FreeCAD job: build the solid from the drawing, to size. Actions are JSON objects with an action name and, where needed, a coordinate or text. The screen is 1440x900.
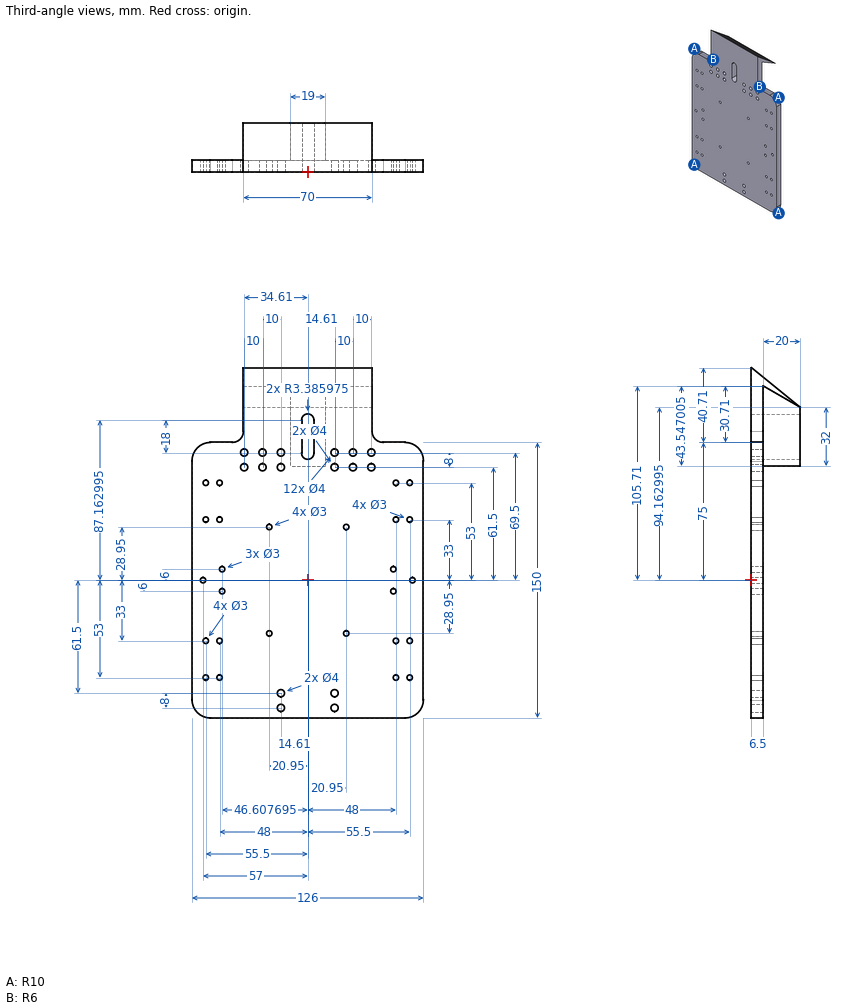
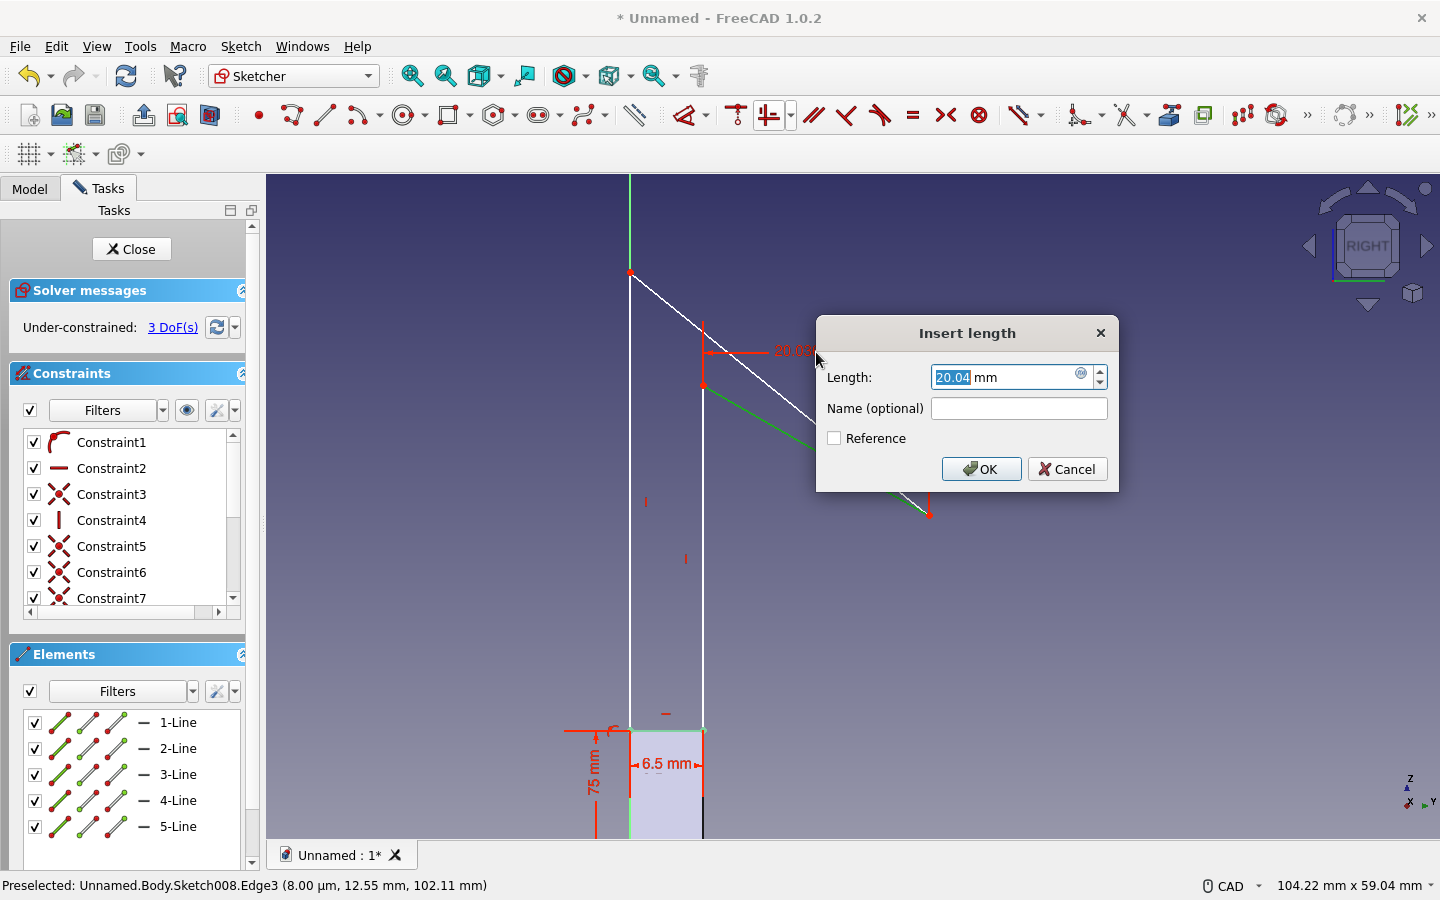
{"action": "type", "text": "20"}
{"action": "key", "text": "Return"}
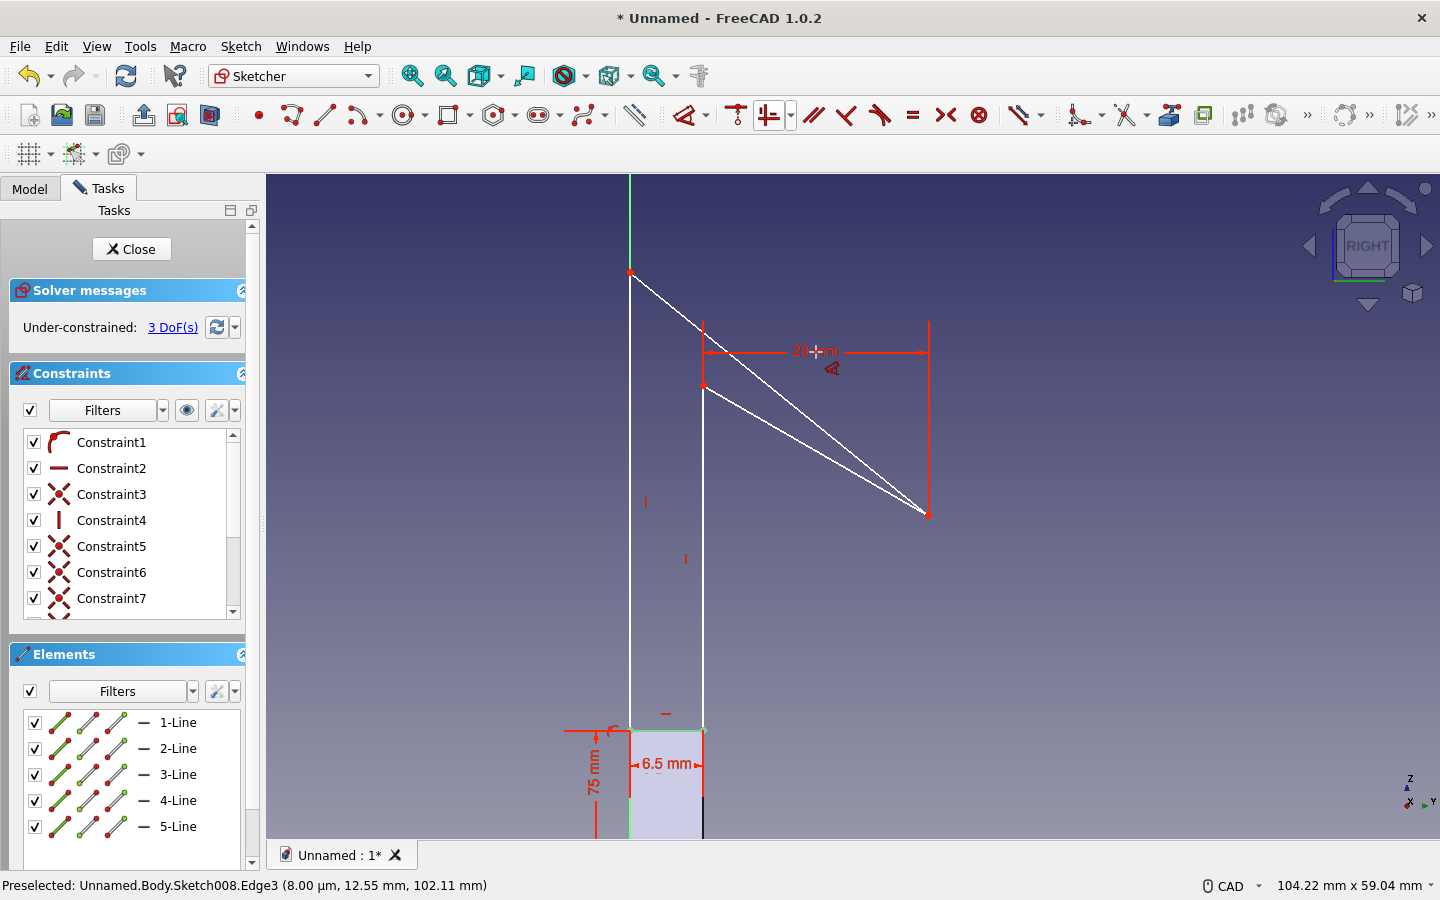
{"action": "left_click", "coordinate": [703, 627]}
{"action": "left_click", "coordinate": [669, 558]}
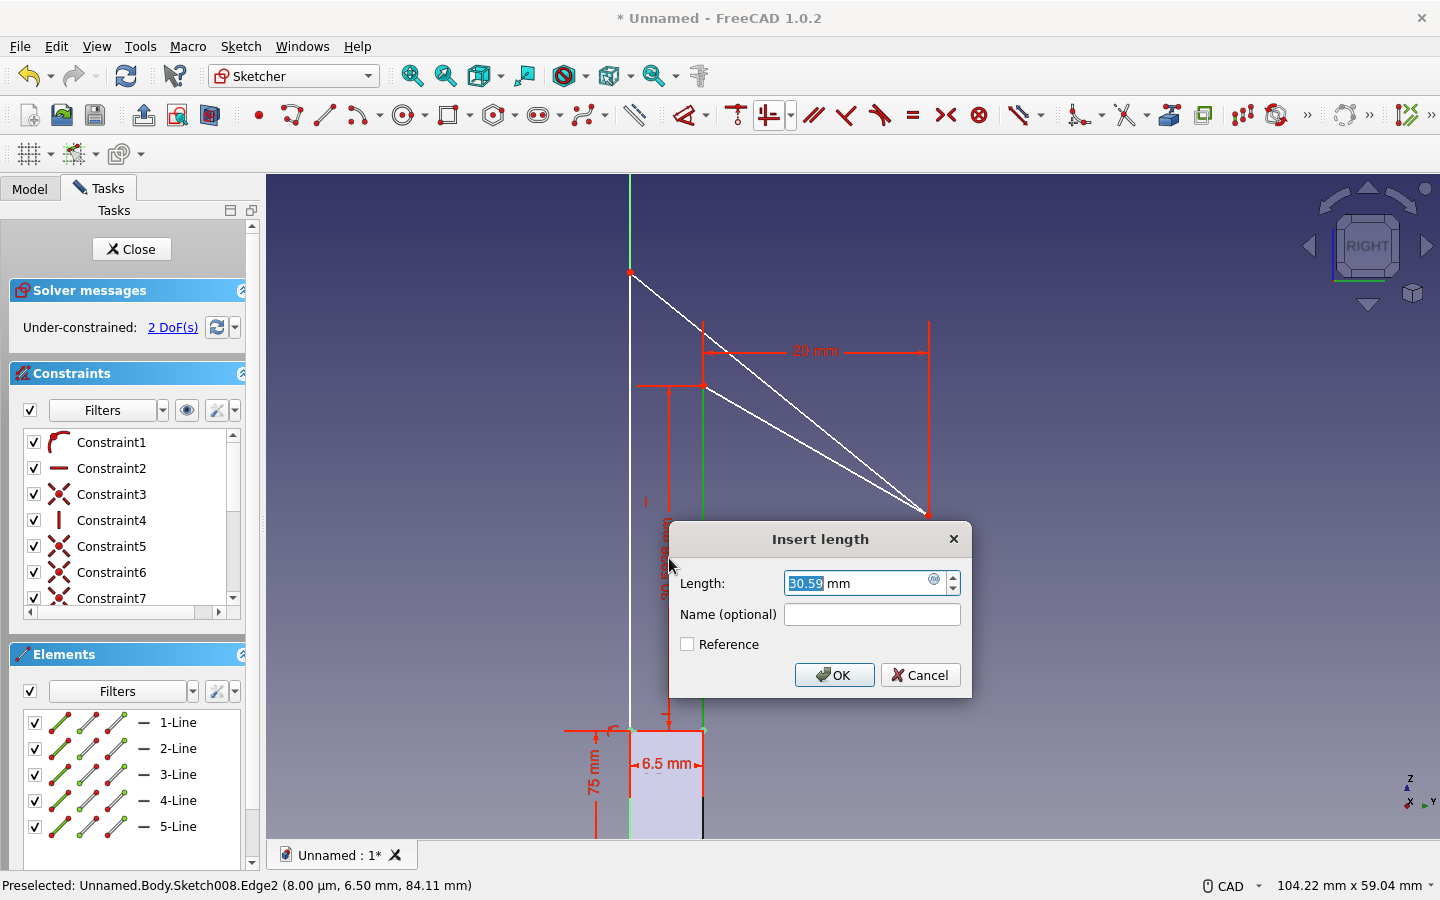
{"action": "type", "text": "30.71"}
{"action": "key", "text": "Return"}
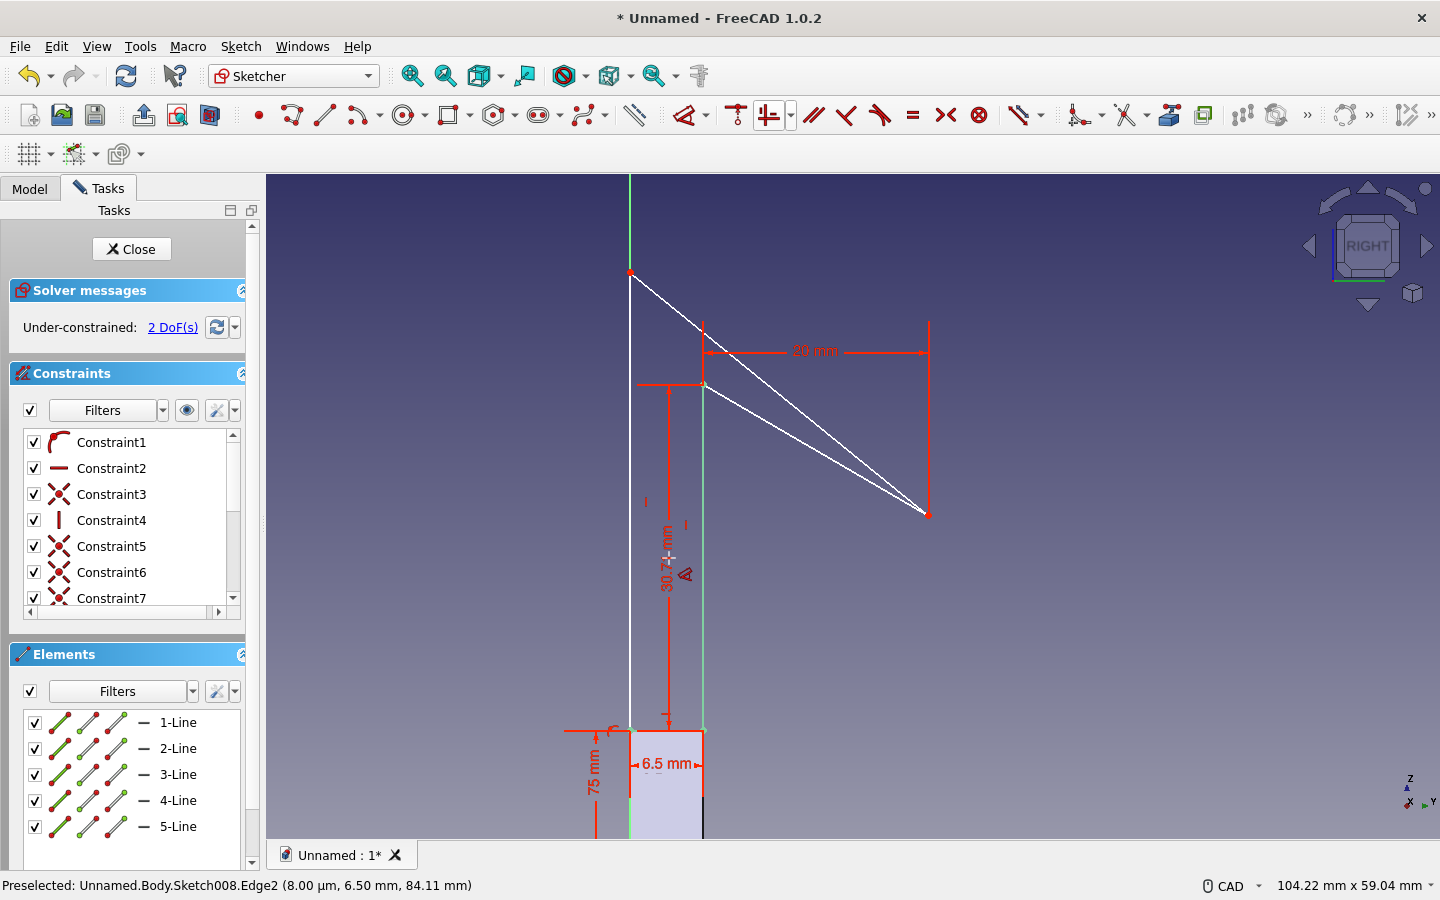
{"action": "left_click", "coordinate": [630, 410]}
{"action": "left_click", "coordinate": [596, 502]}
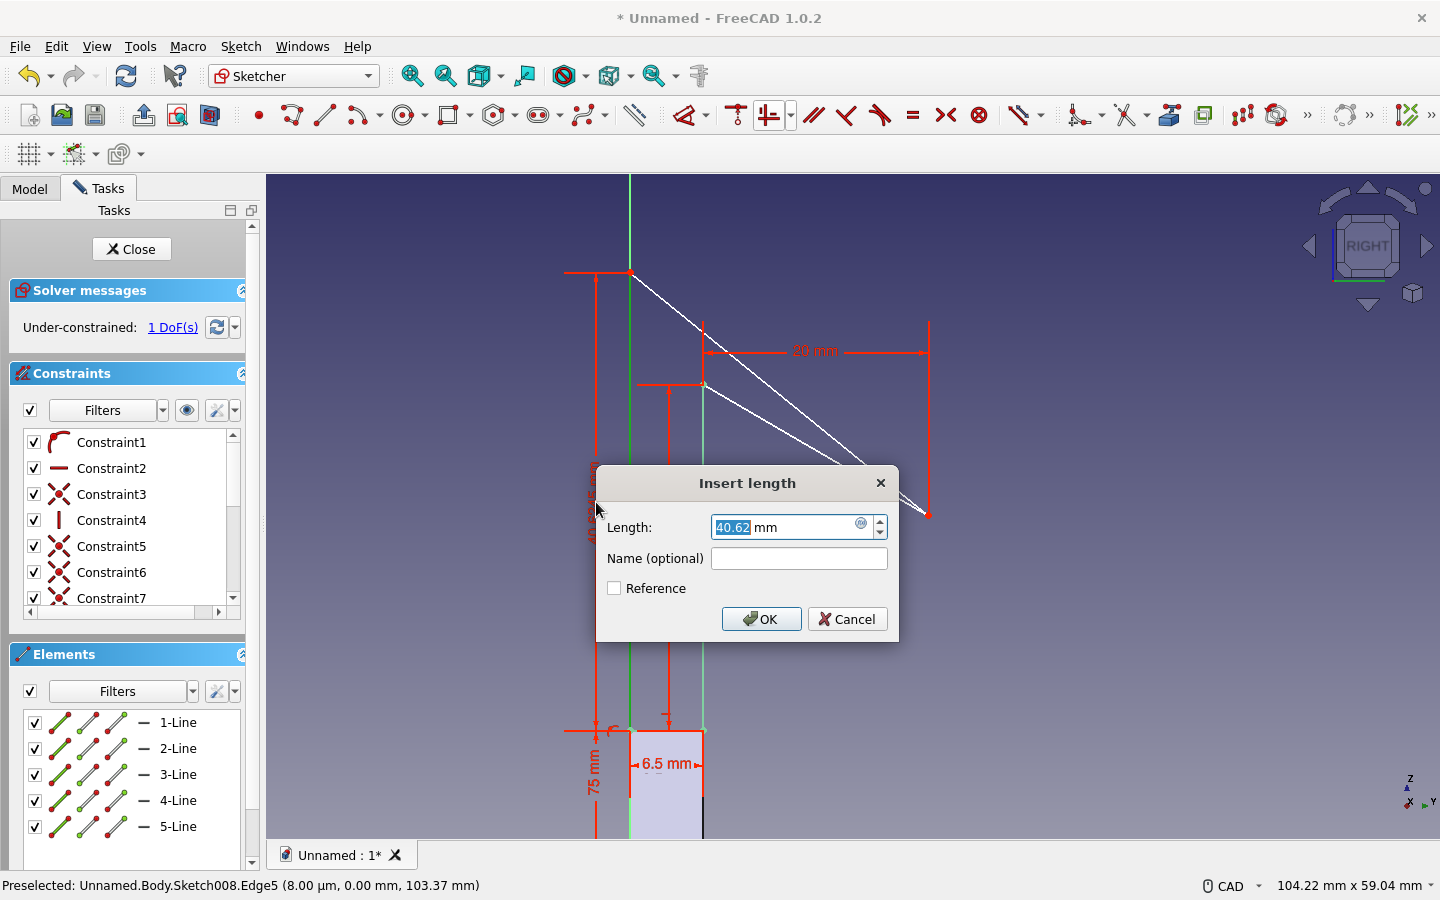
{"action": "type", "text": "40.71"}
{"action": "key", "text": "Return"}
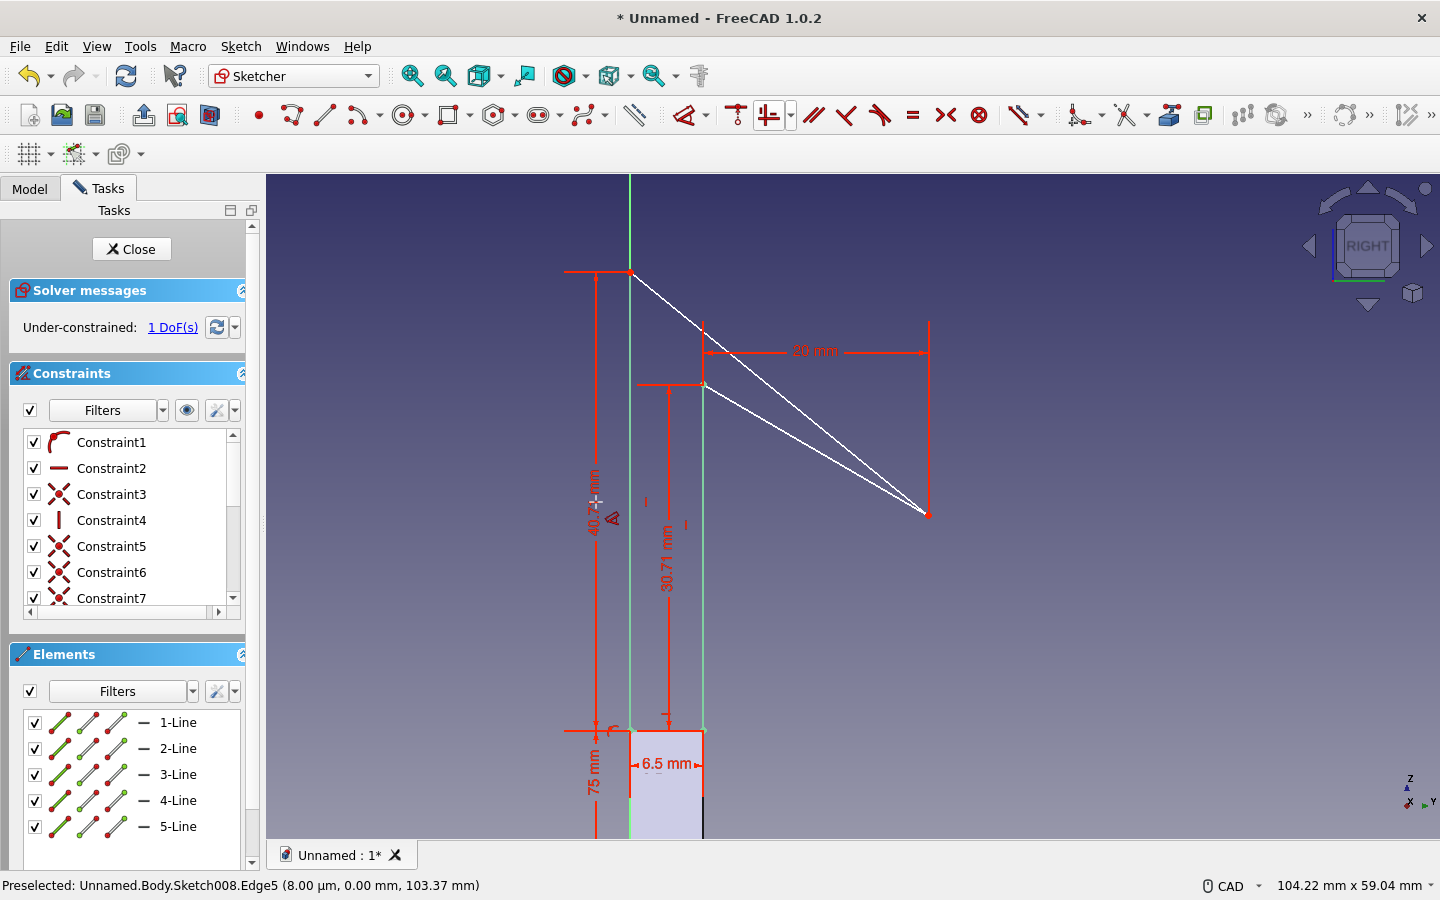
{"action": "left_click", "coordinate": [929, 516]}
{"action": "left_click", "coordinate": [963, 664]}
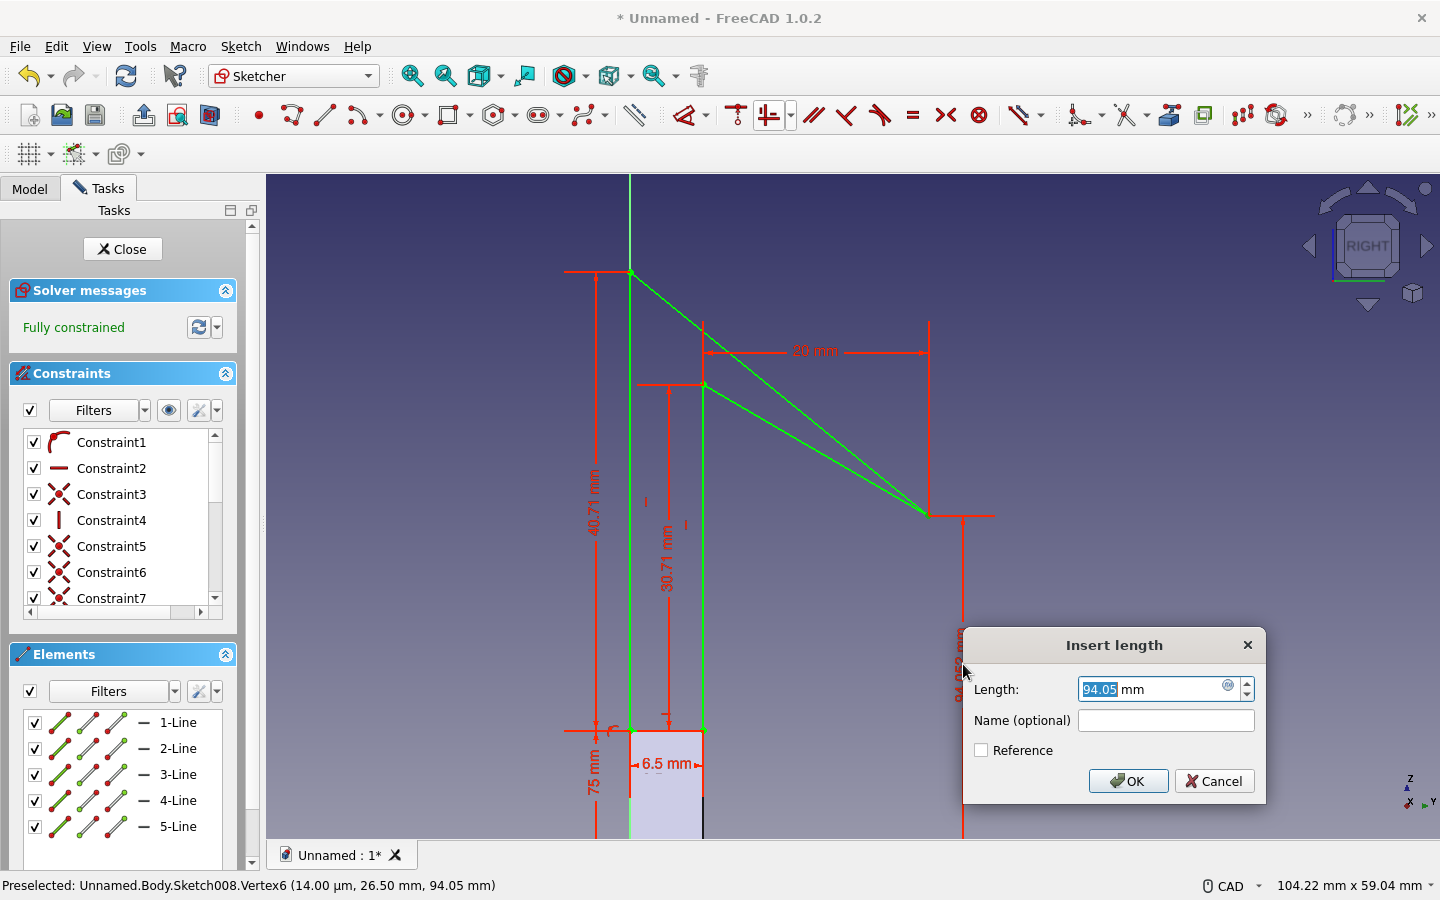
{"action": "type", "text": "94.162995"}
{"action": "key", "text": "Return"}
{"action": "key", "text": "Escape"}